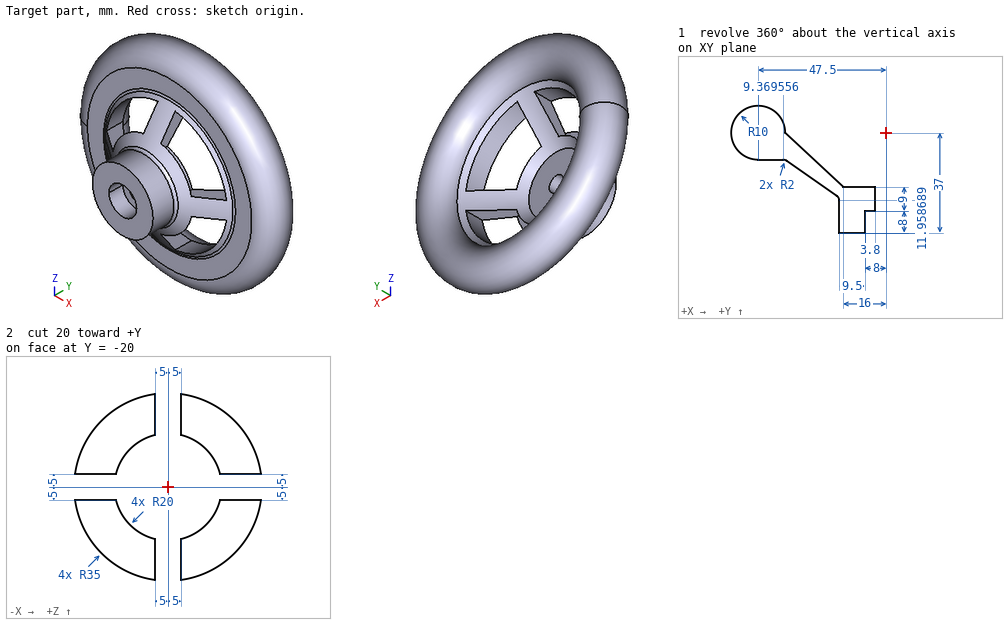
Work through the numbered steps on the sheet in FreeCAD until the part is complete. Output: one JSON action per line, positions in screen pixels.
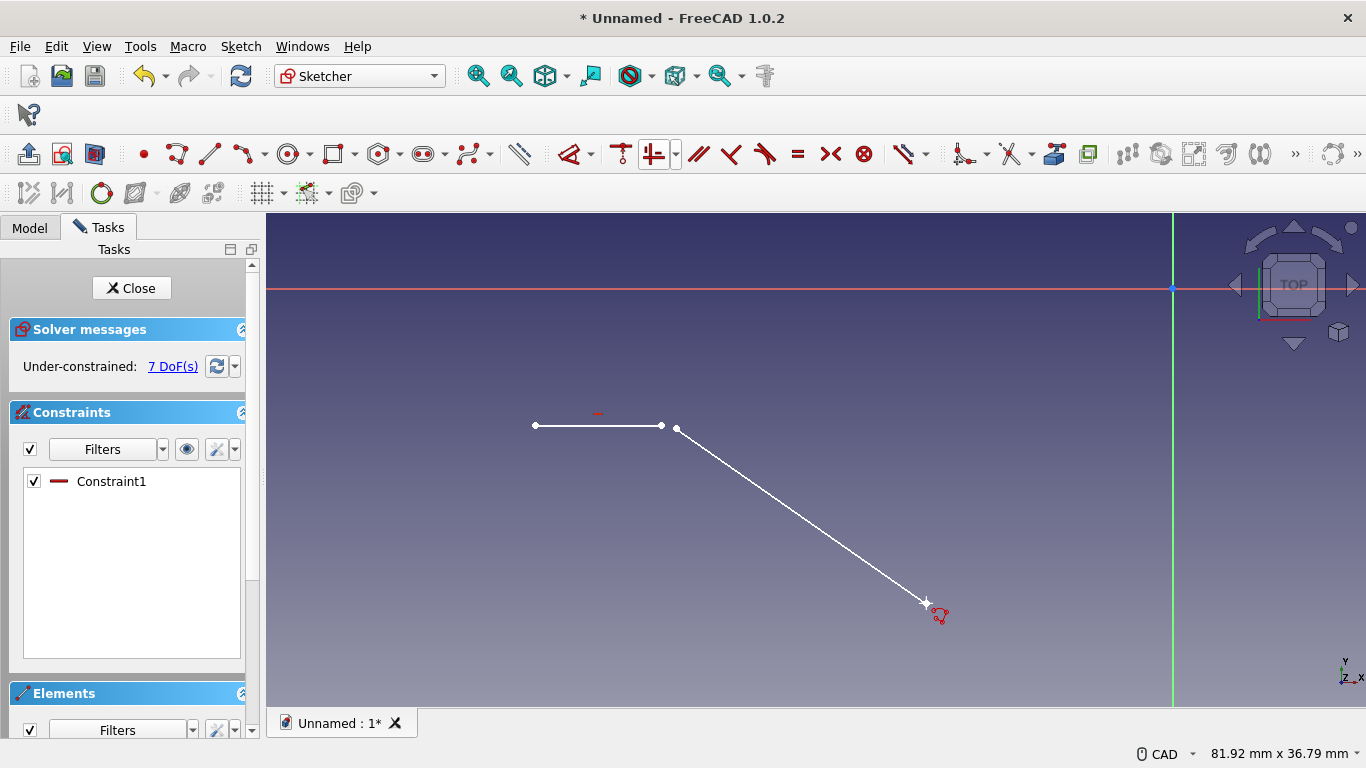
{"action": "left_click", "coordinate": [938, 625]}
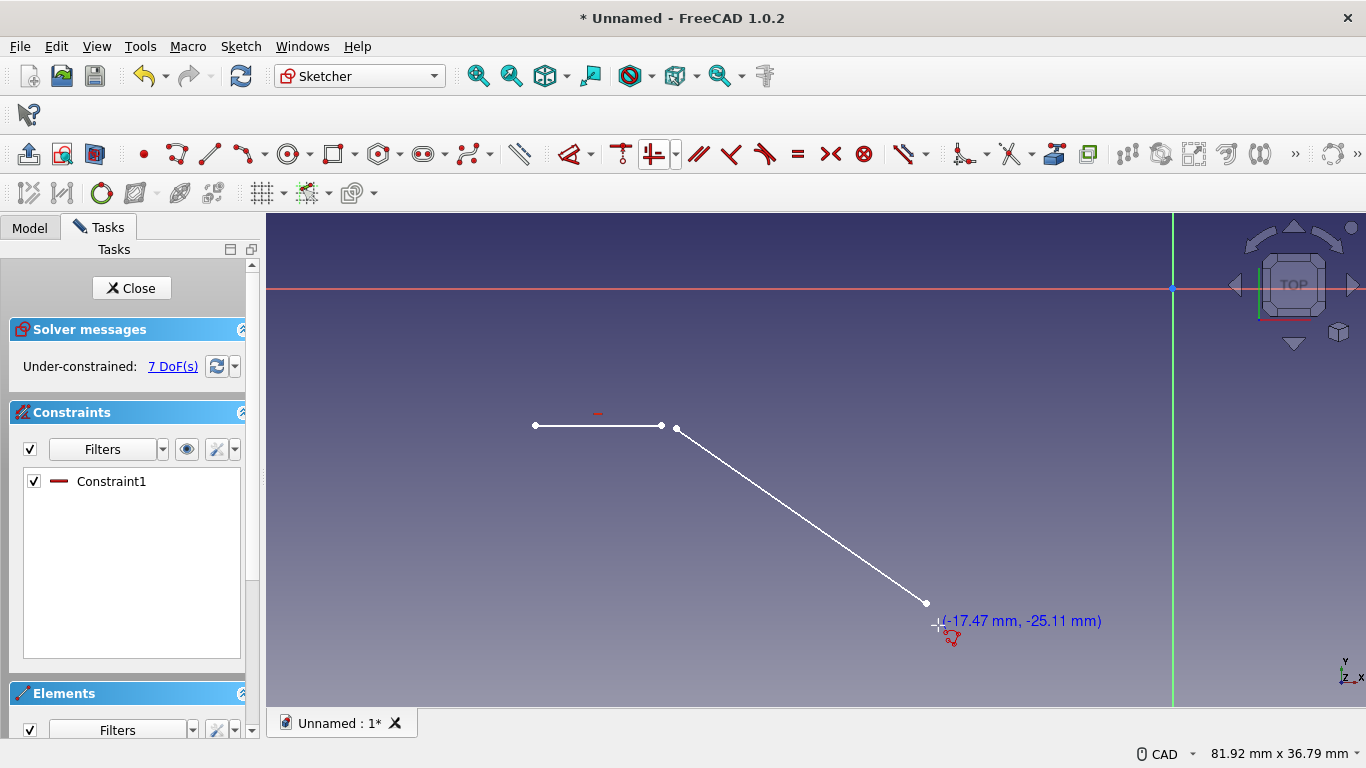
{"action": "scroll", "coordinate": [676, 424], "scroll_direction": "down", "scroll_amount": 3}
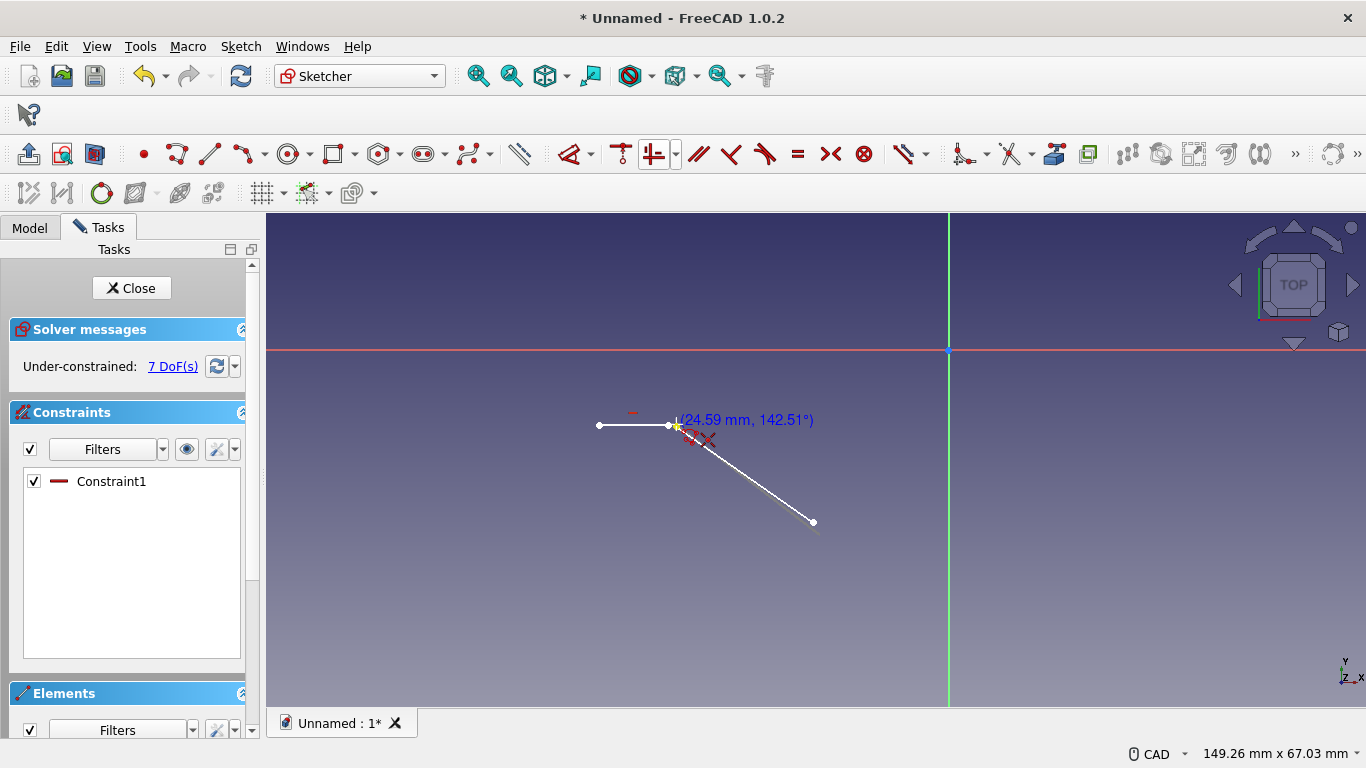
{"action": "left_click", "coordinate": [820, 623]}
{"action": "left_click", "coordinate": [890, 623]}
{"action": "left_click", "coordinate": [890, 564]}
{"action": "left_click", "coordinate": [918, 564]}
{"action": "left_click", "coordinate": [918, 497]}
{"action": "left_click", "coordinate": [831, 497]}
{"action": "left_click", "coordinate": [672, 350]}
{"action": "right_click", "coordinate": [672, 350]}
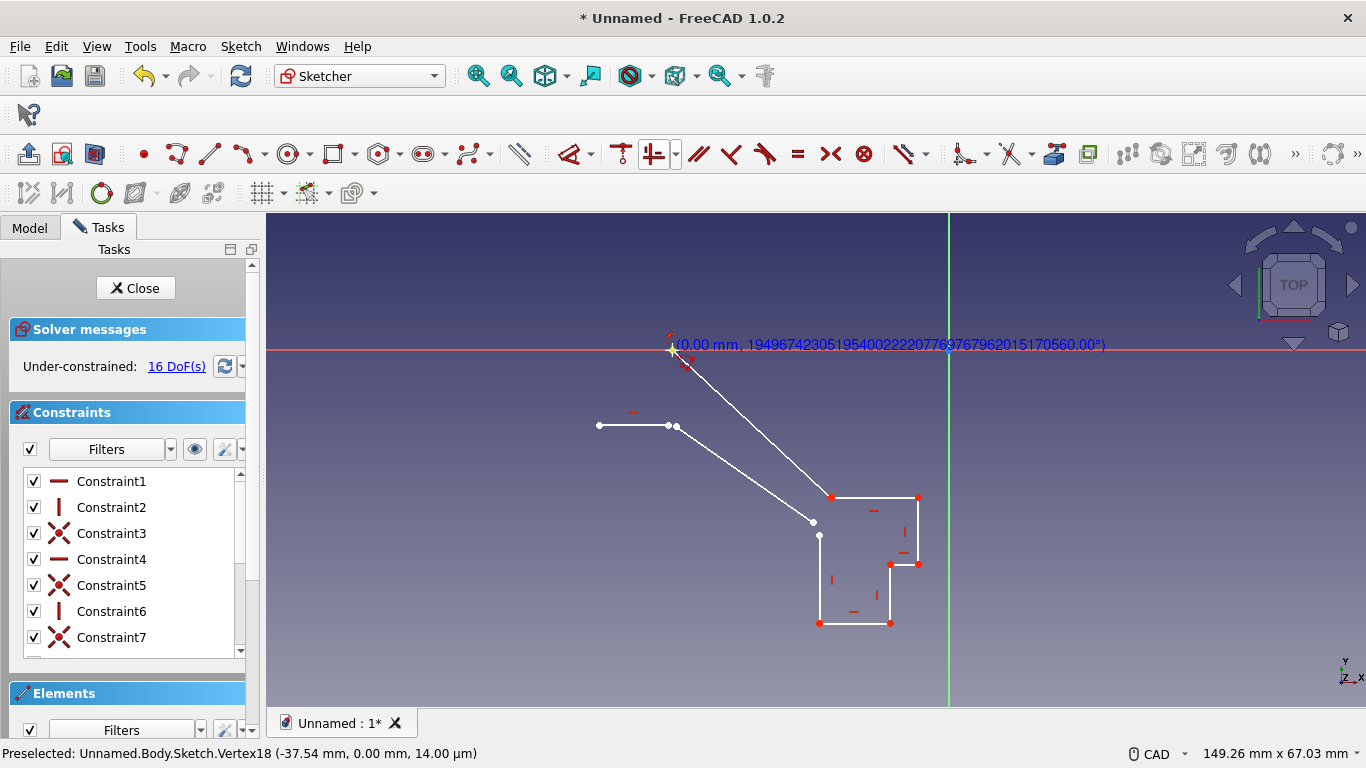
{"action": "left_click", "coordinate": [242, 154]}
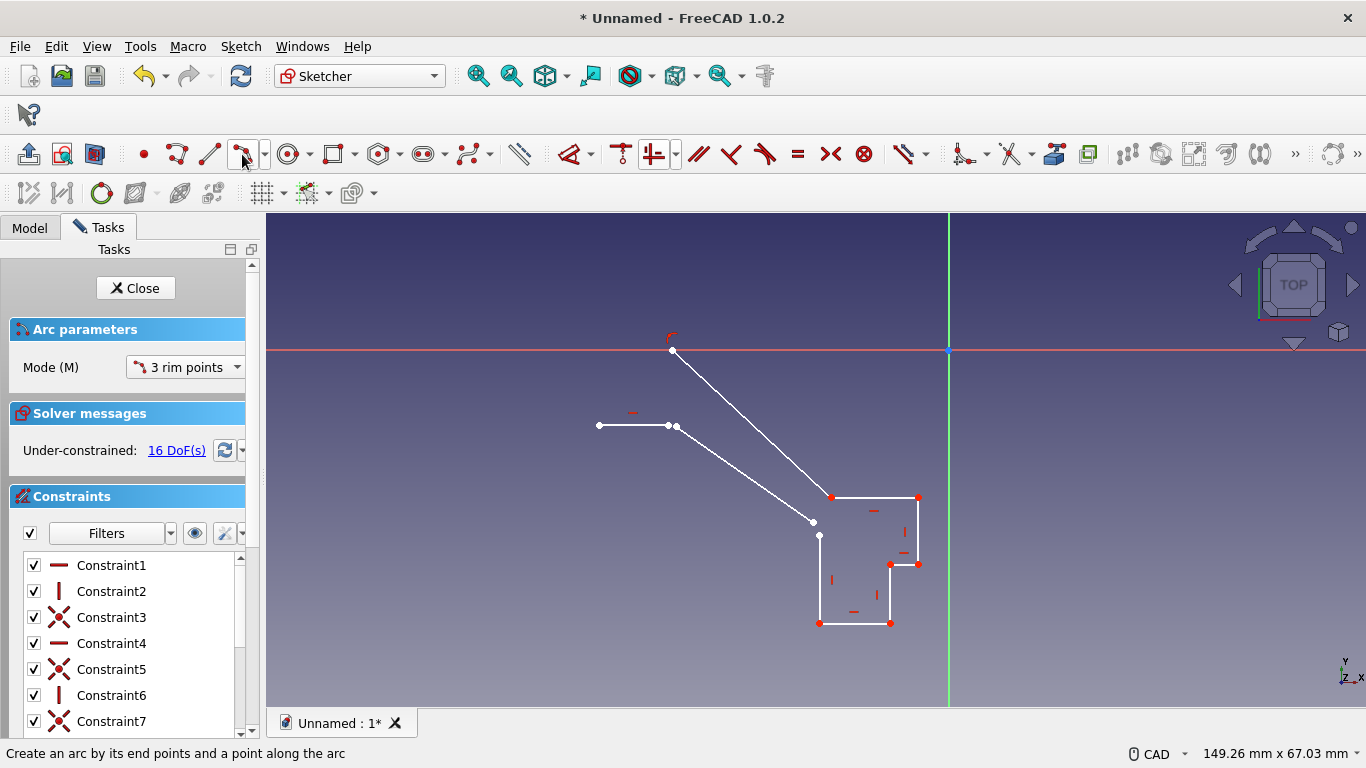
{"action": "scroll", "coordinate": [668, 424], "scroll_direction": "up", "scroll_amount": 3}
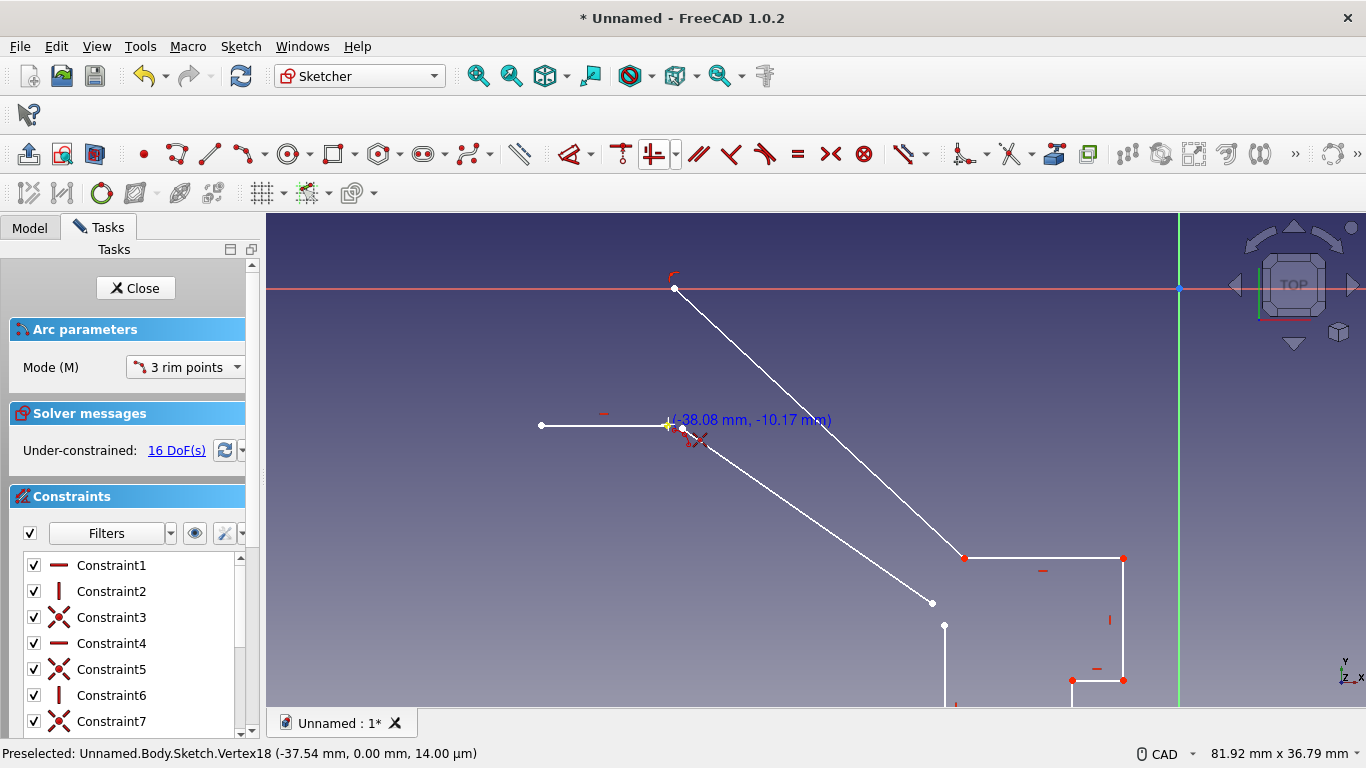
{"action": "left_click", "coordinate": [668, 426]}
{"action": "left_click", "coordinate": [683, 429]}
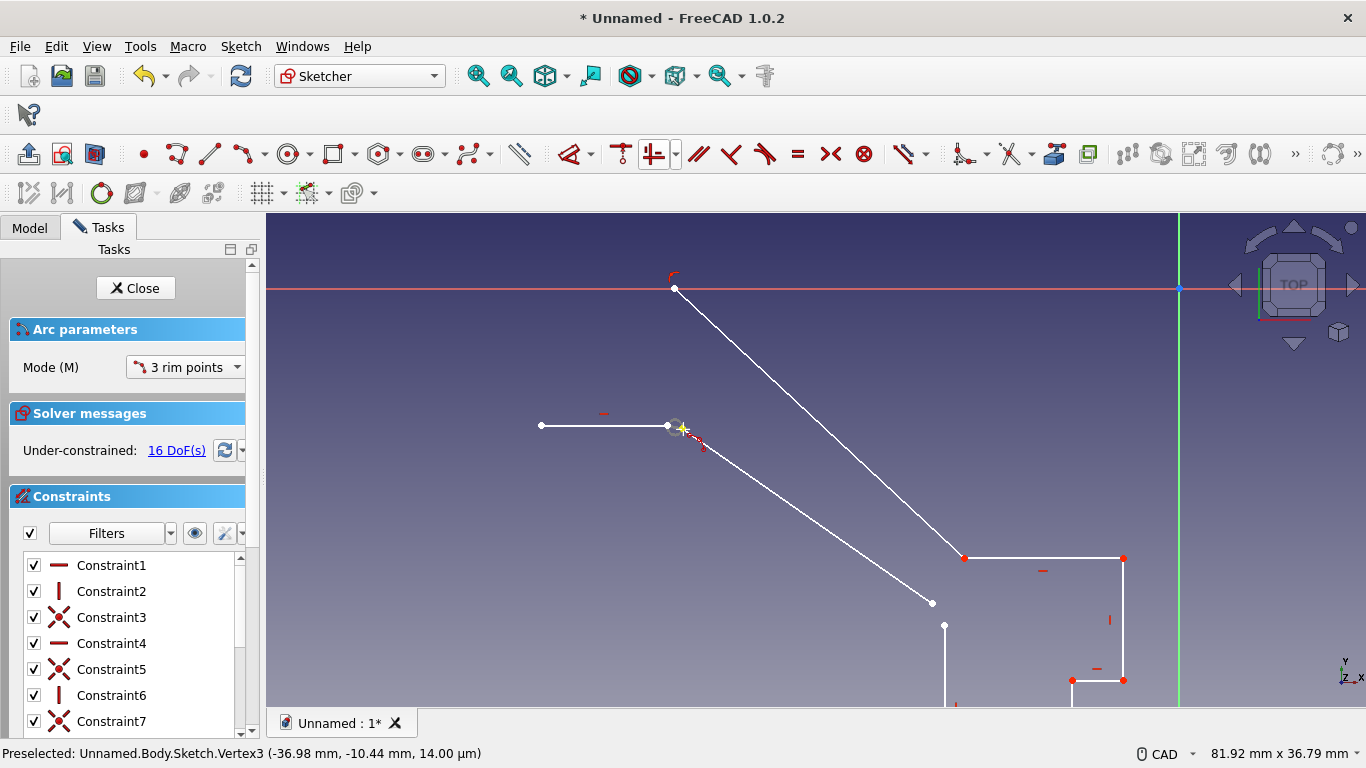
{"action": "scroll", "coordinate": [675, 424], "scroll_direction": "up", "scroll_amount": 13}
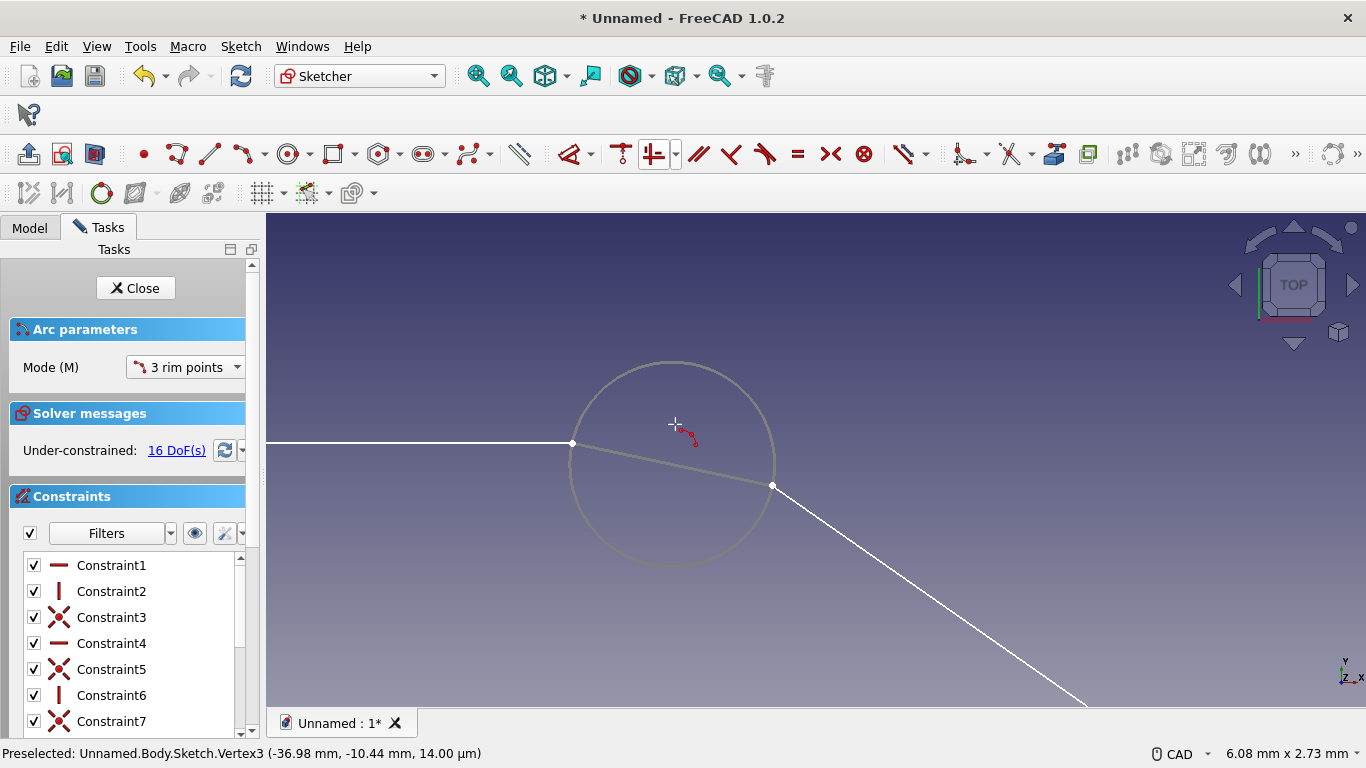
{"action": "left_click", "coordinate": [672, 424]}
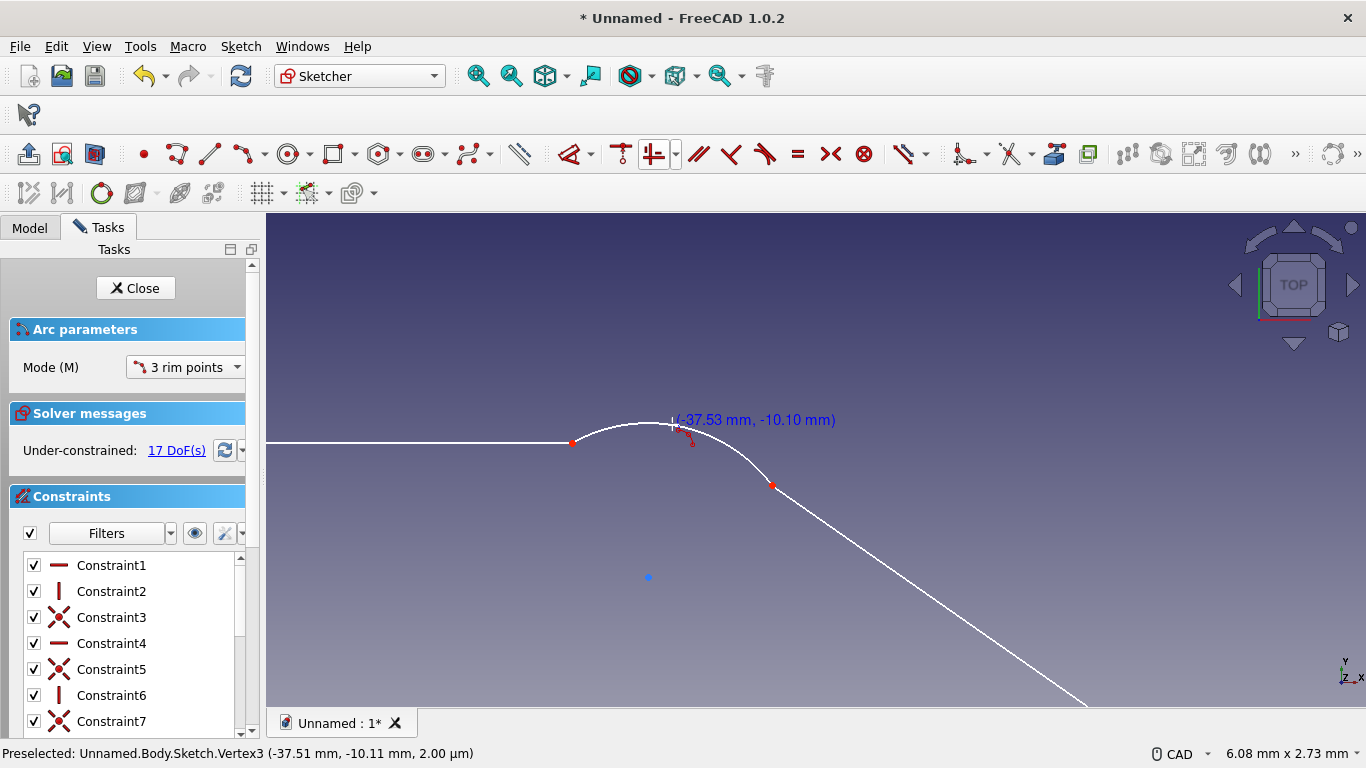
{"action": "scroll", "coordinate": [672, 424], "scroll_direction": "down", "scroll_amount": 16}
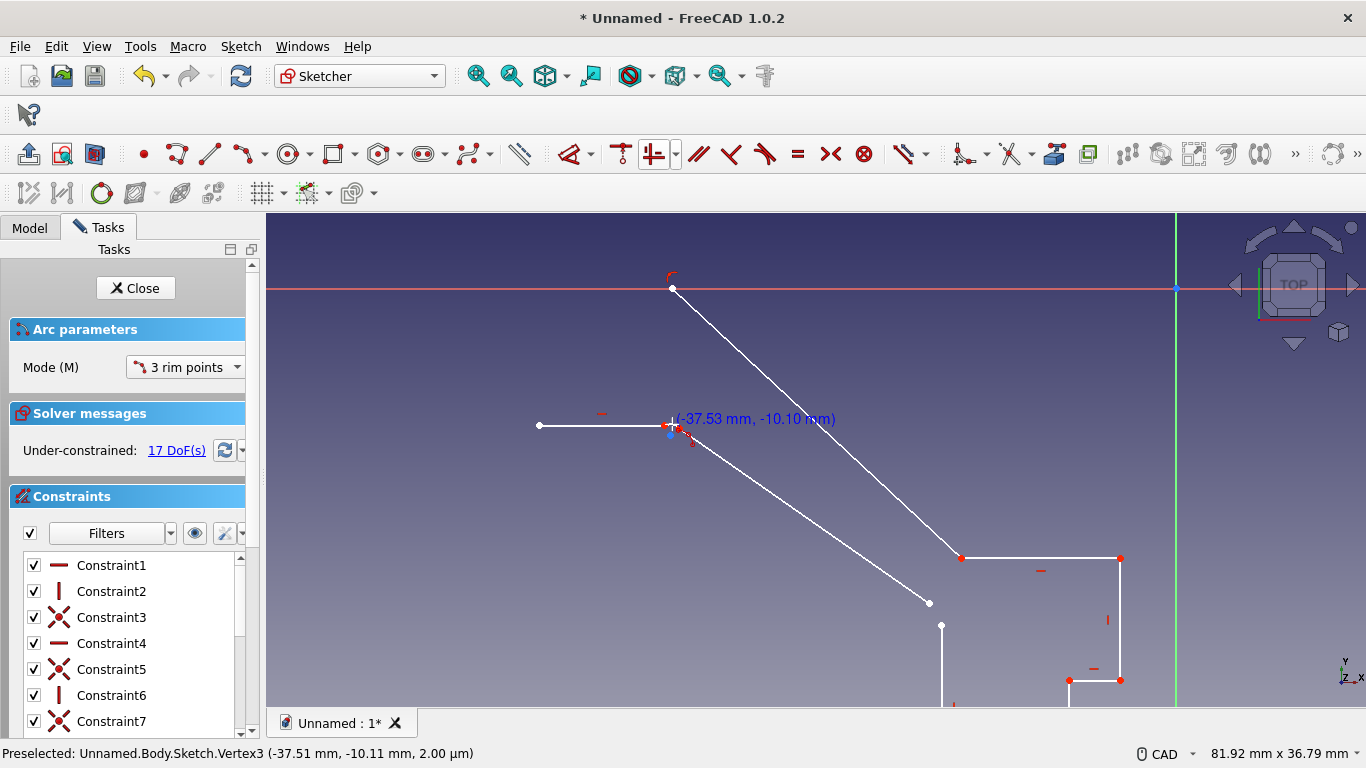
{"action": "left_click", "coordinate": [814, 523]}
{"action": "left_click", "coordinate": [820, 535]}